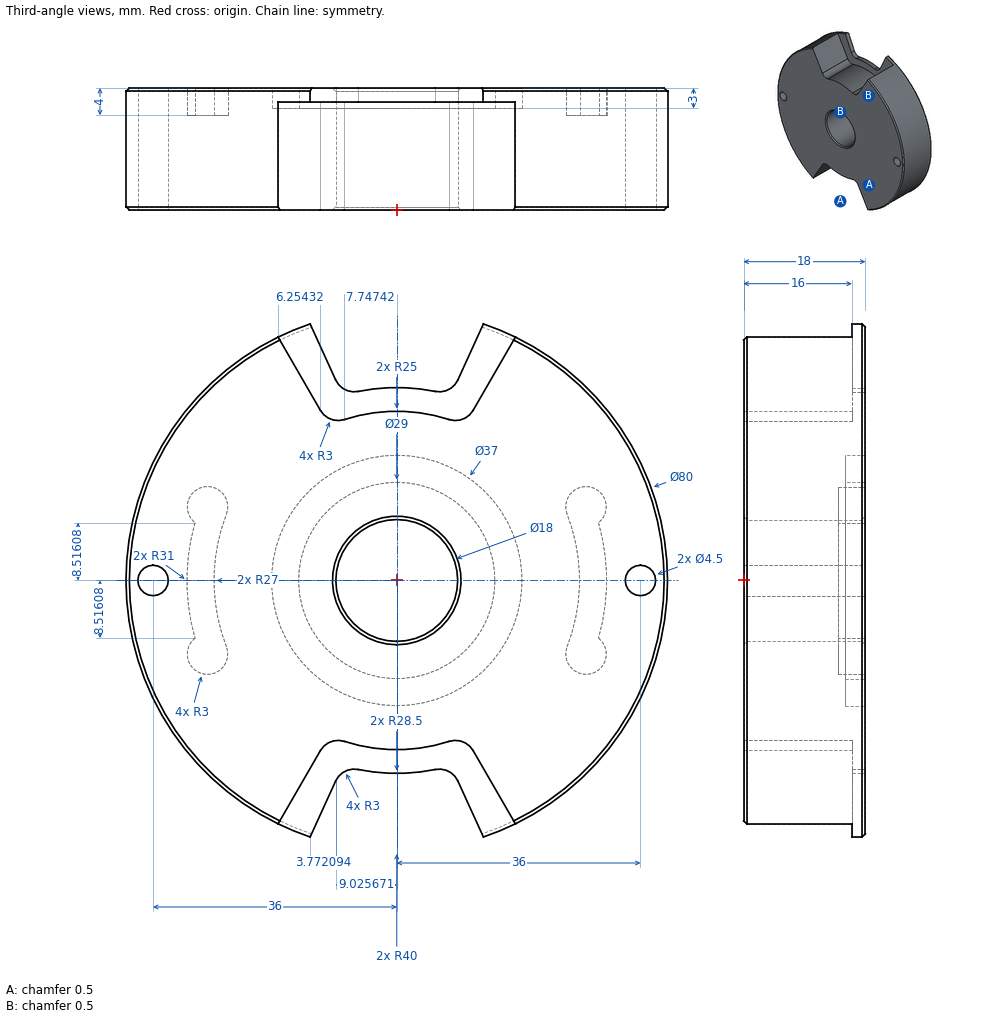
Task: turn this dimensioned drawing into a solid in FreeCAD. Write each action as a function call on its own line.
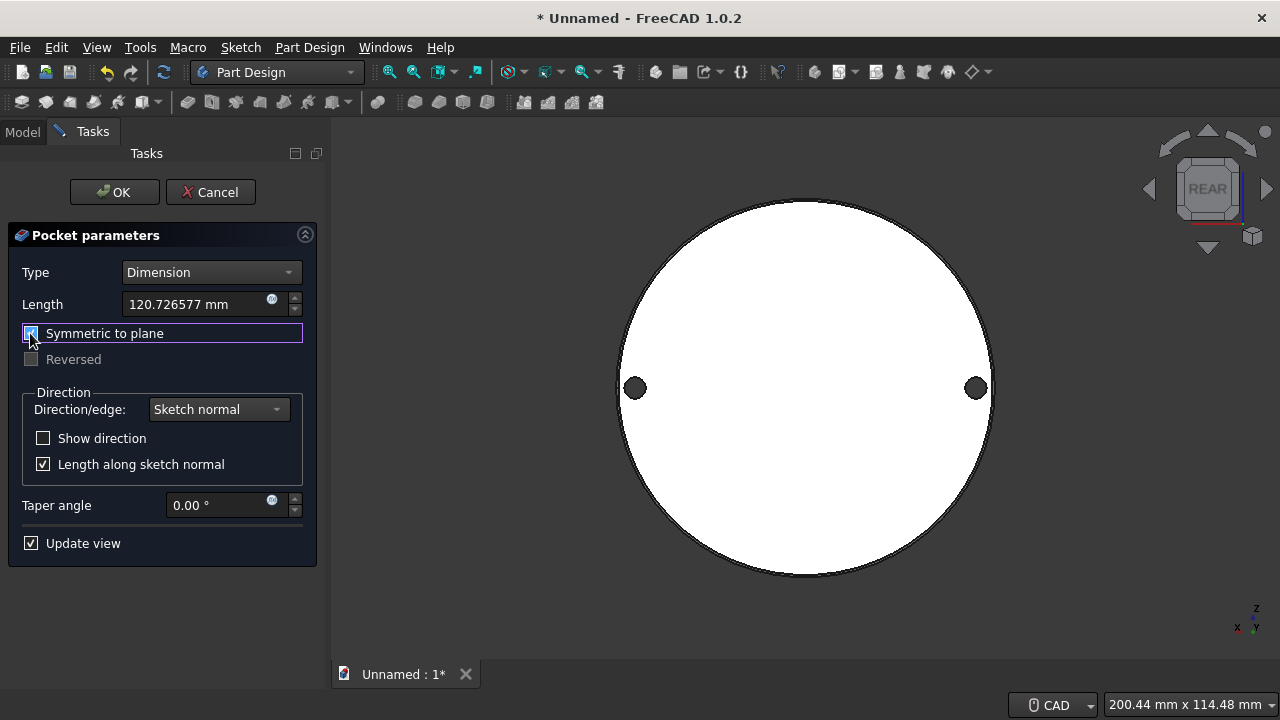
click(115, 192)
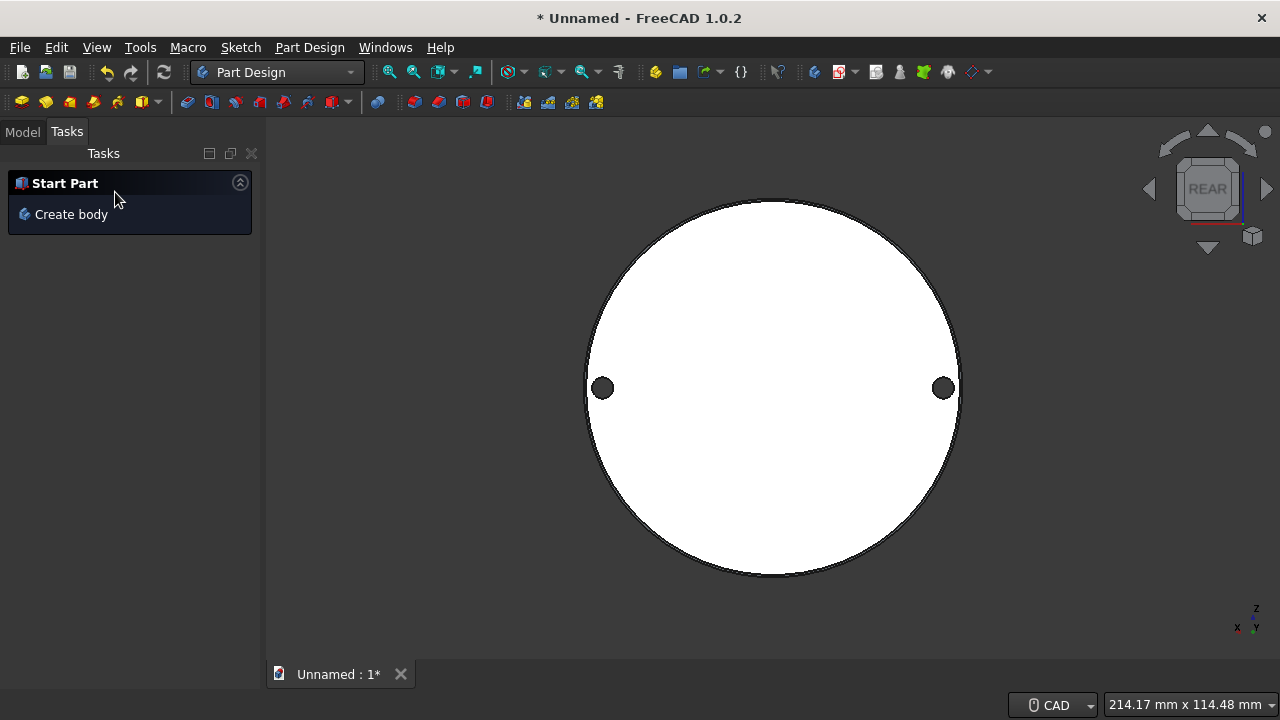
click(773, 387)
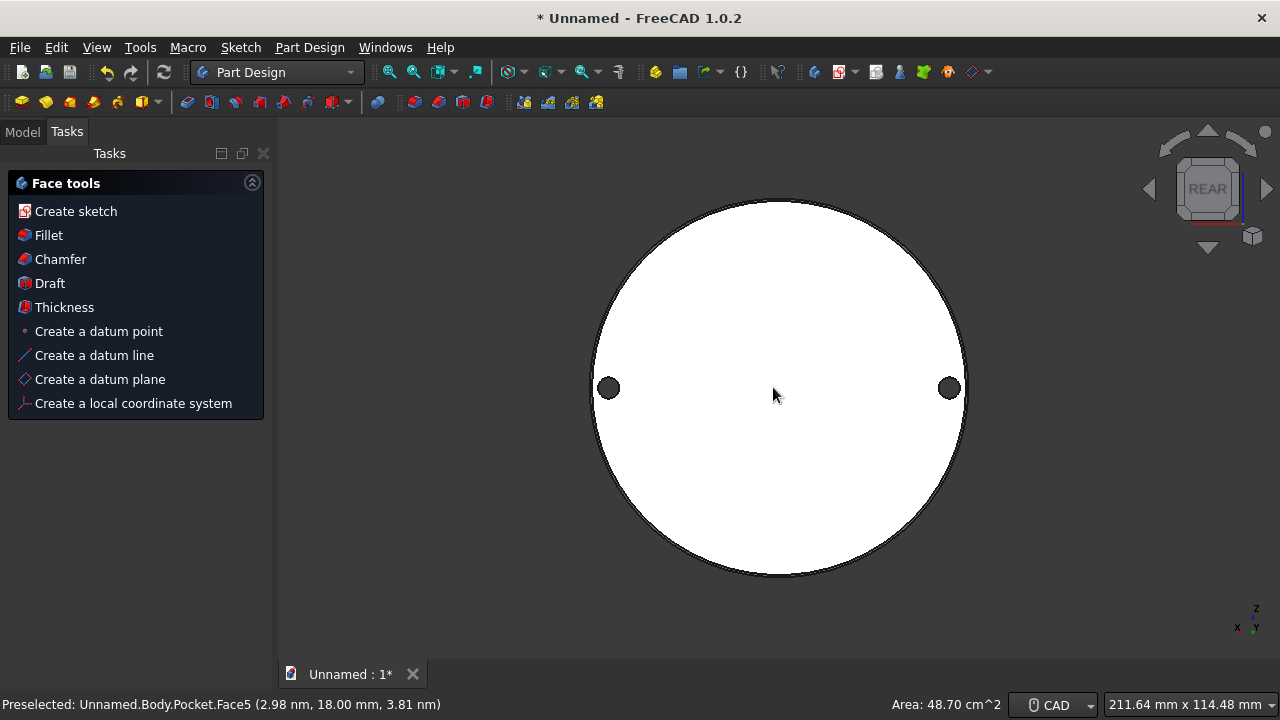
click(840, 72)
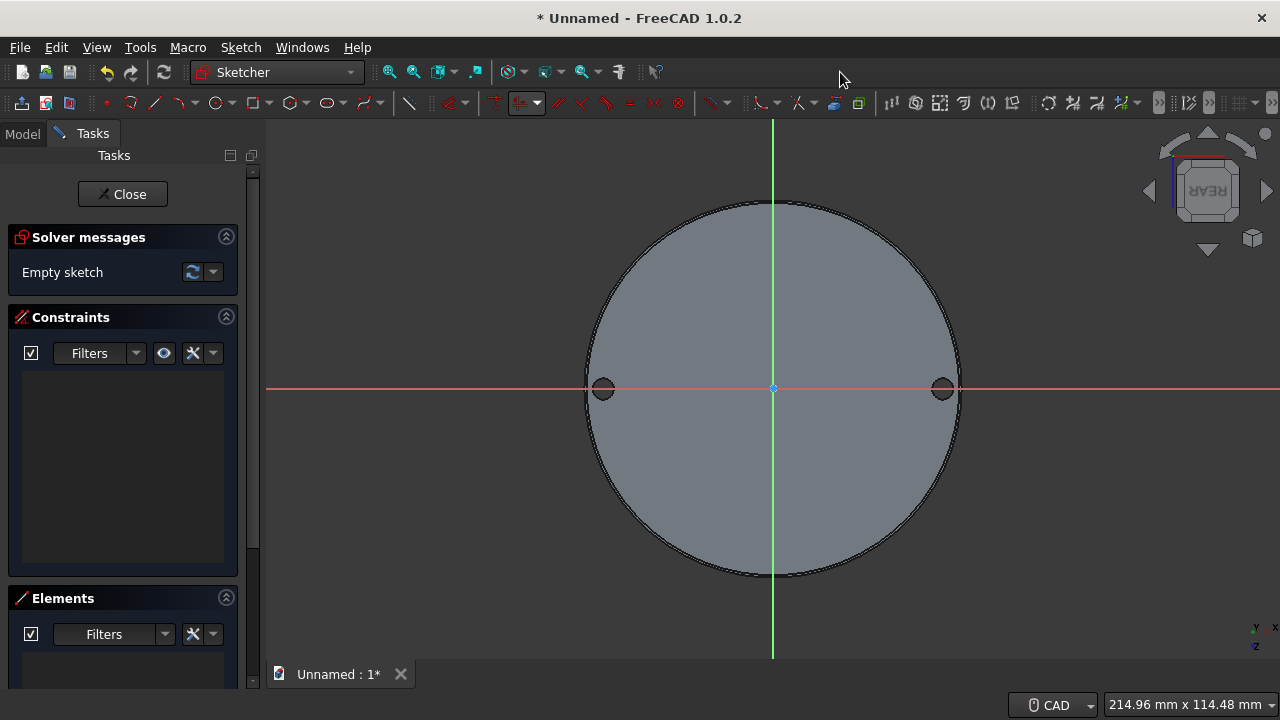
scroll(856, 389, up, 3)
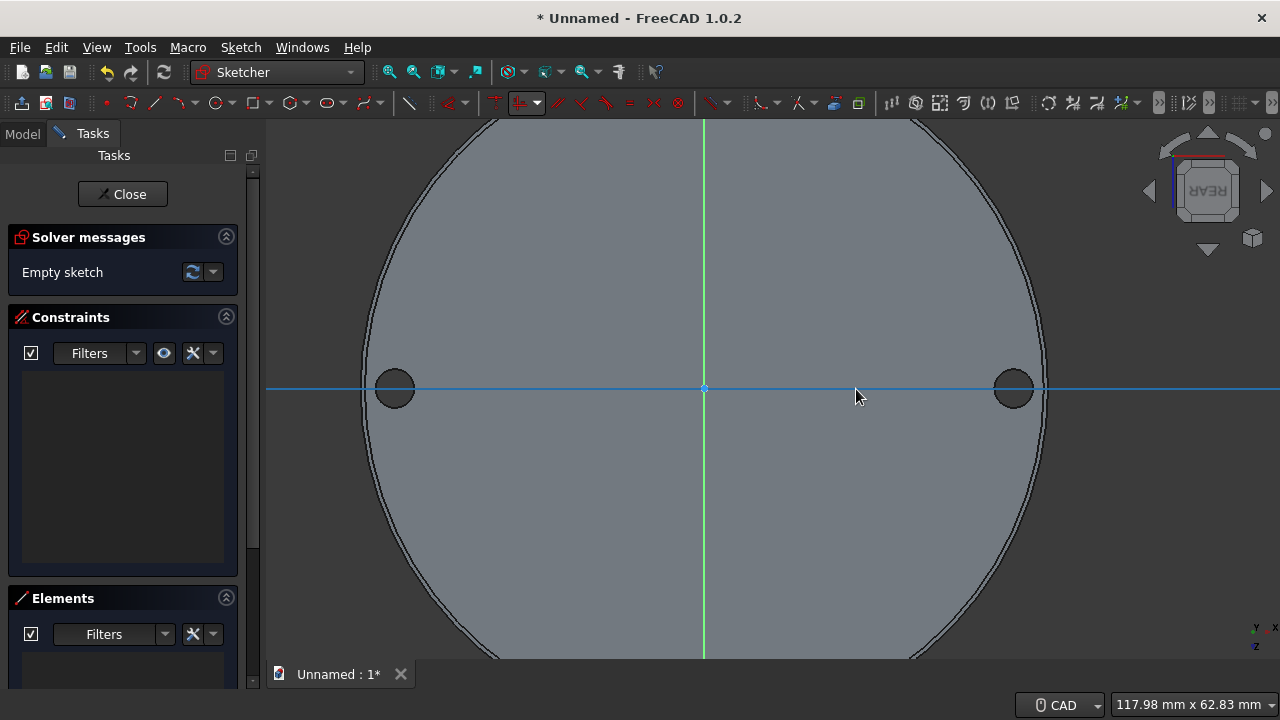
click(180, 104)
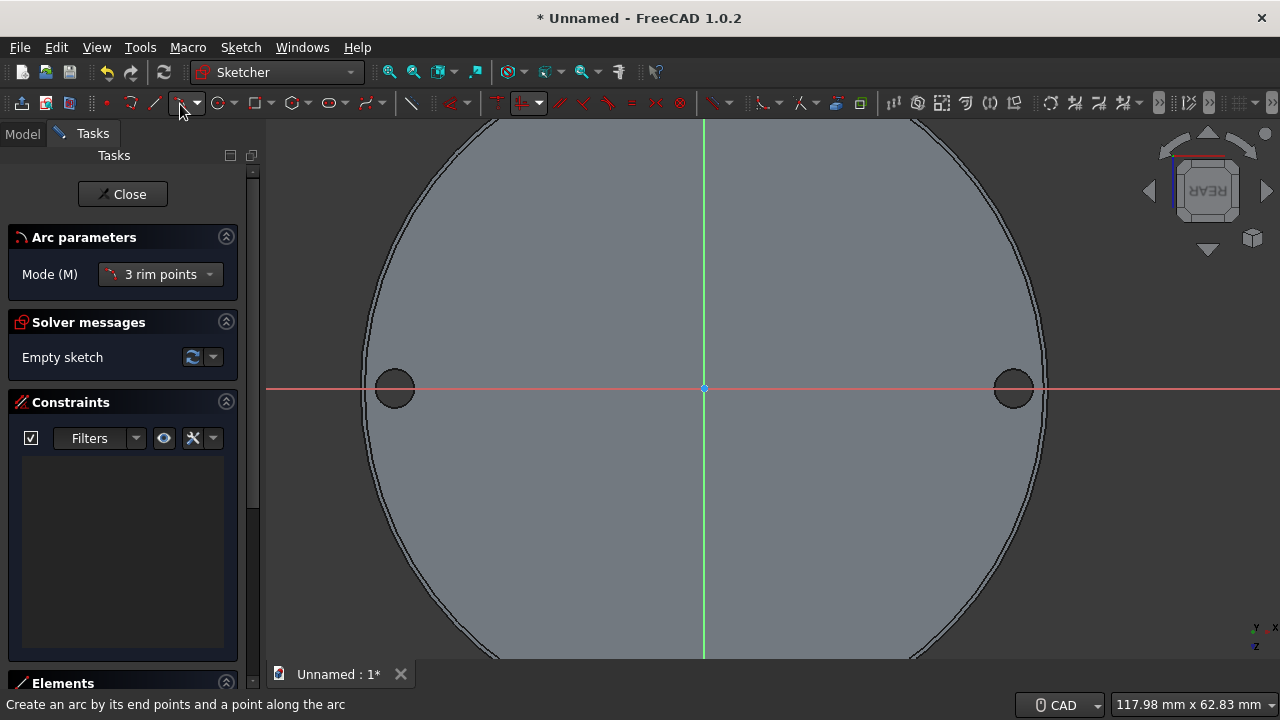
click(488, 473)
click(488, 304)
click(473, 371)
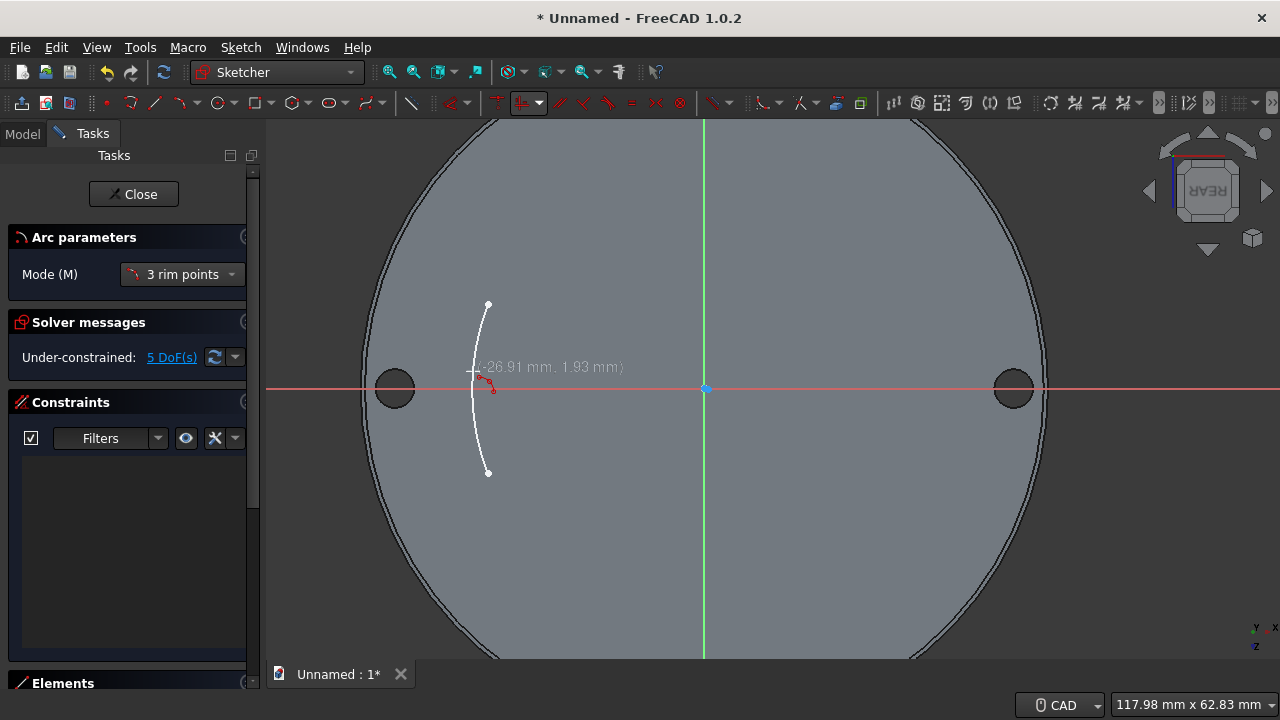
click(488, 305)
click(448, 315)
click(457, 270)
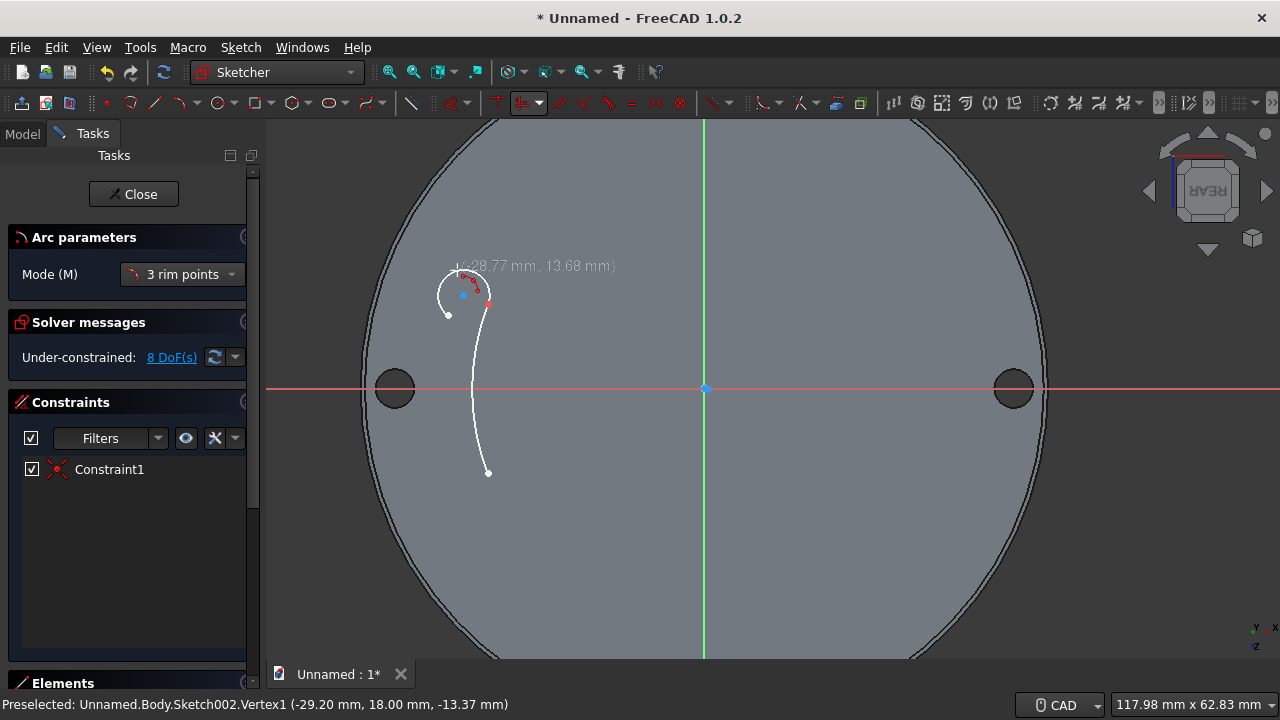
click(448, 316)
click(448, 462)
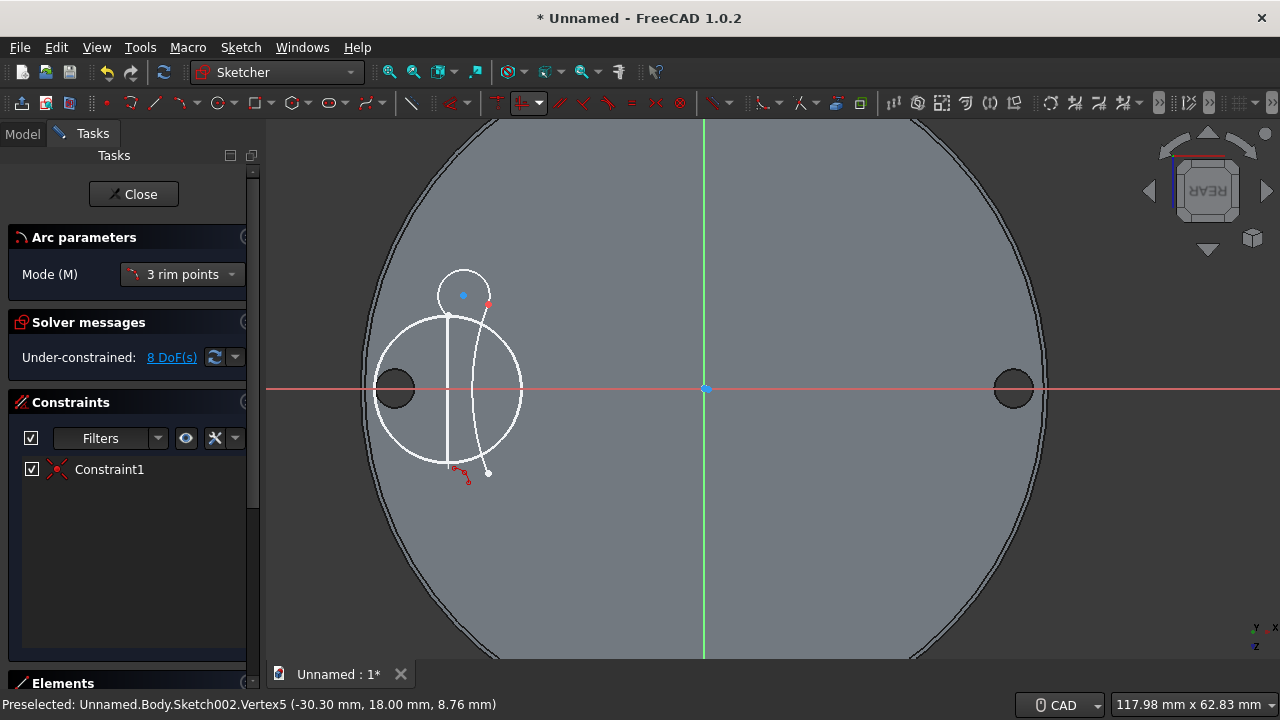
scroll(438, 374, up, 3)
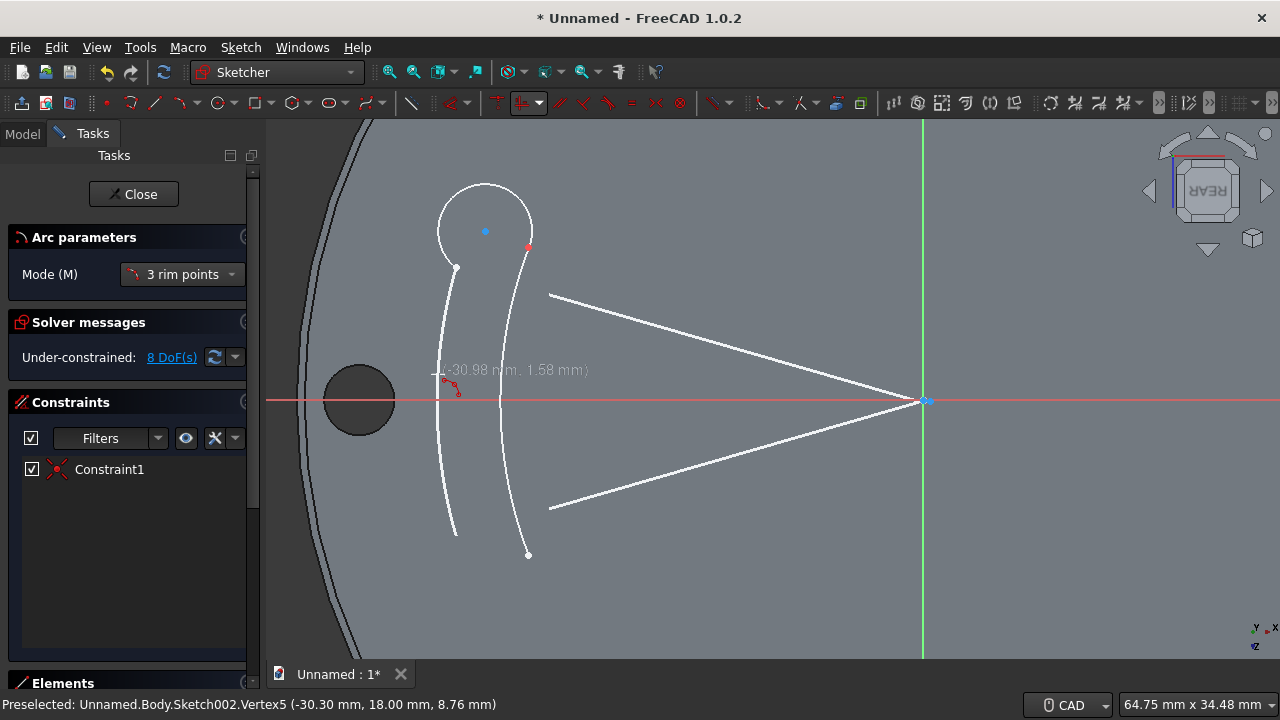
click(438, 373)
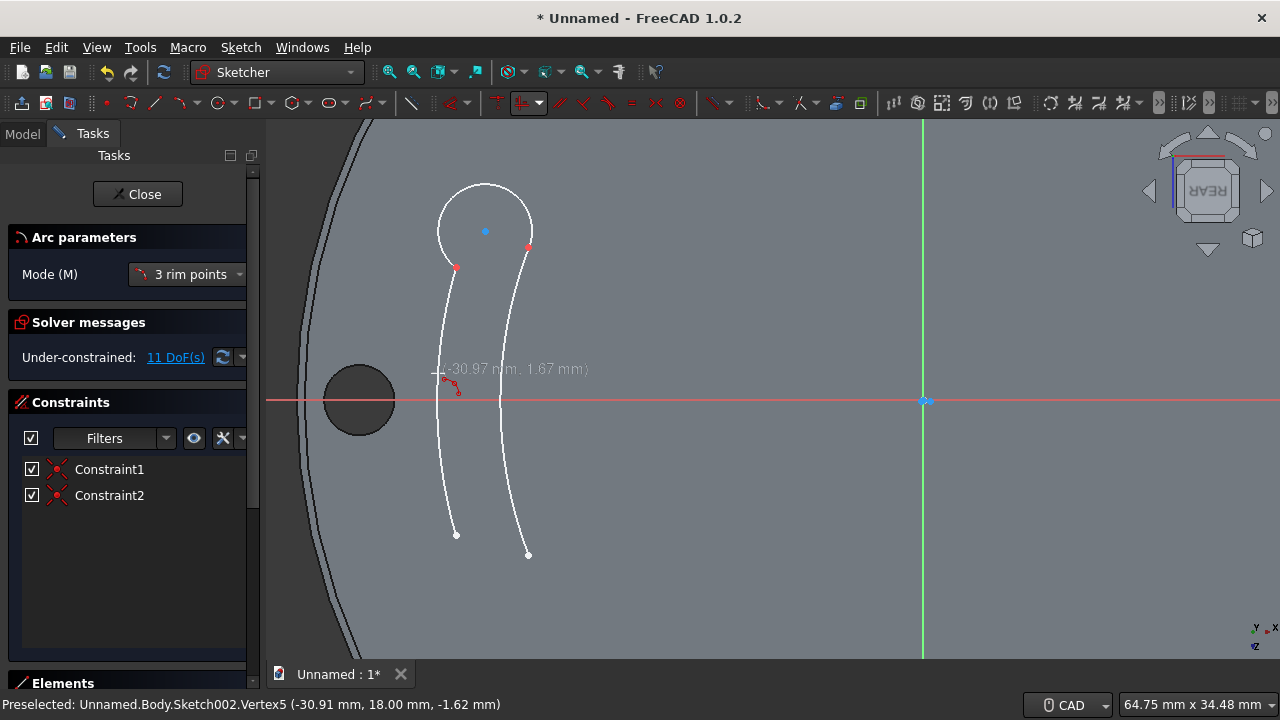
click(456, 536)
click(529, 556)
click(473, 616)